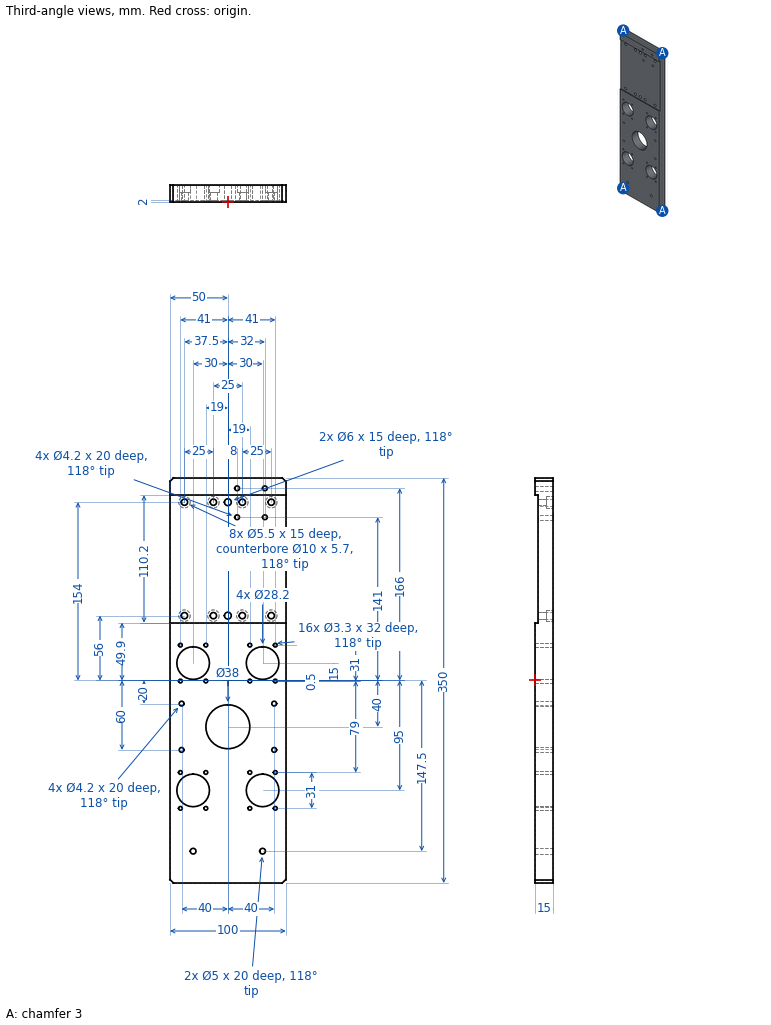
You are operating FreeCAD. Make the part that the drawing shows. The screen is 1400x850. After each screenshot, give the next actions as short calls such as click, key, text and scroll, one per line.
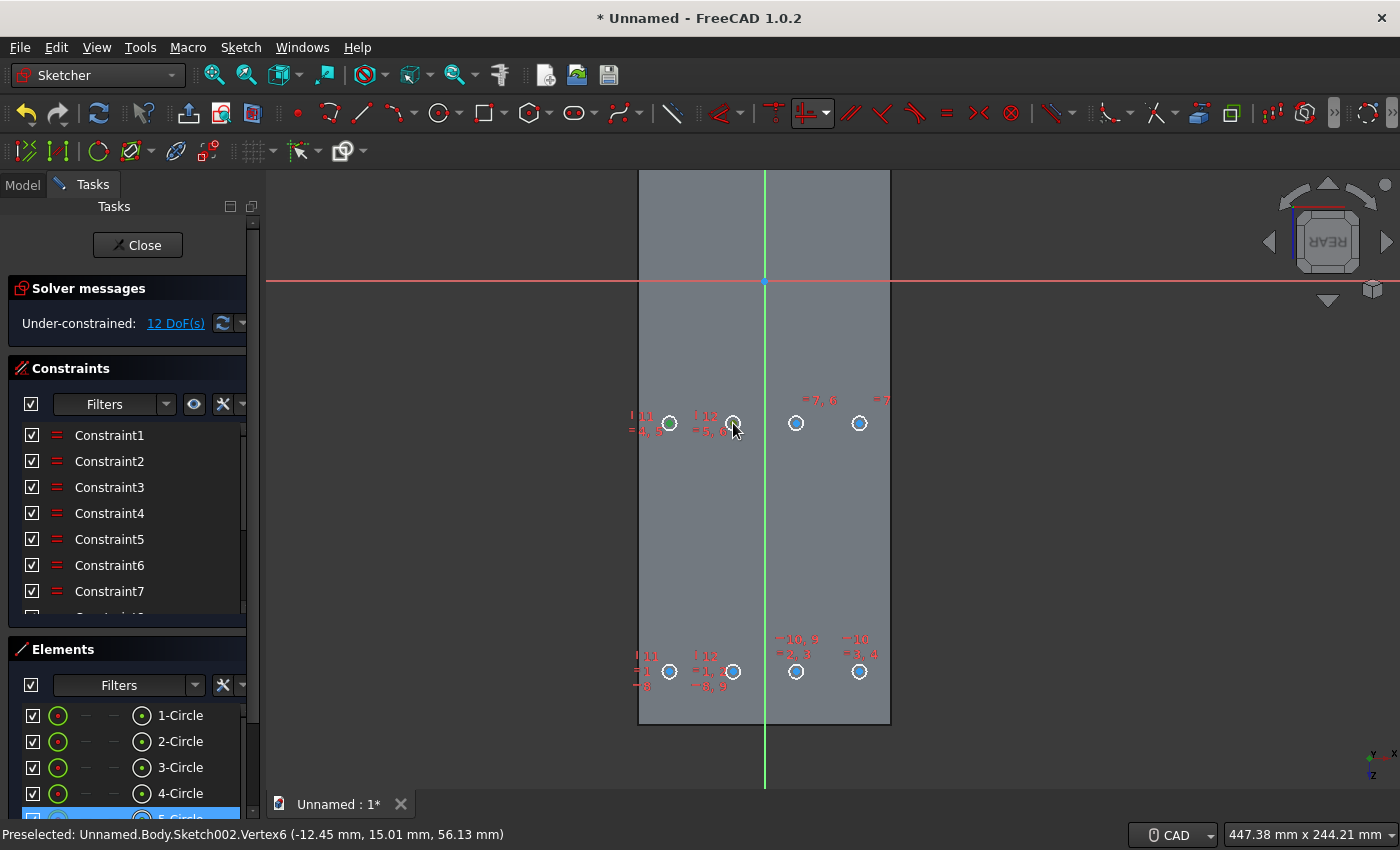
click(828, 114)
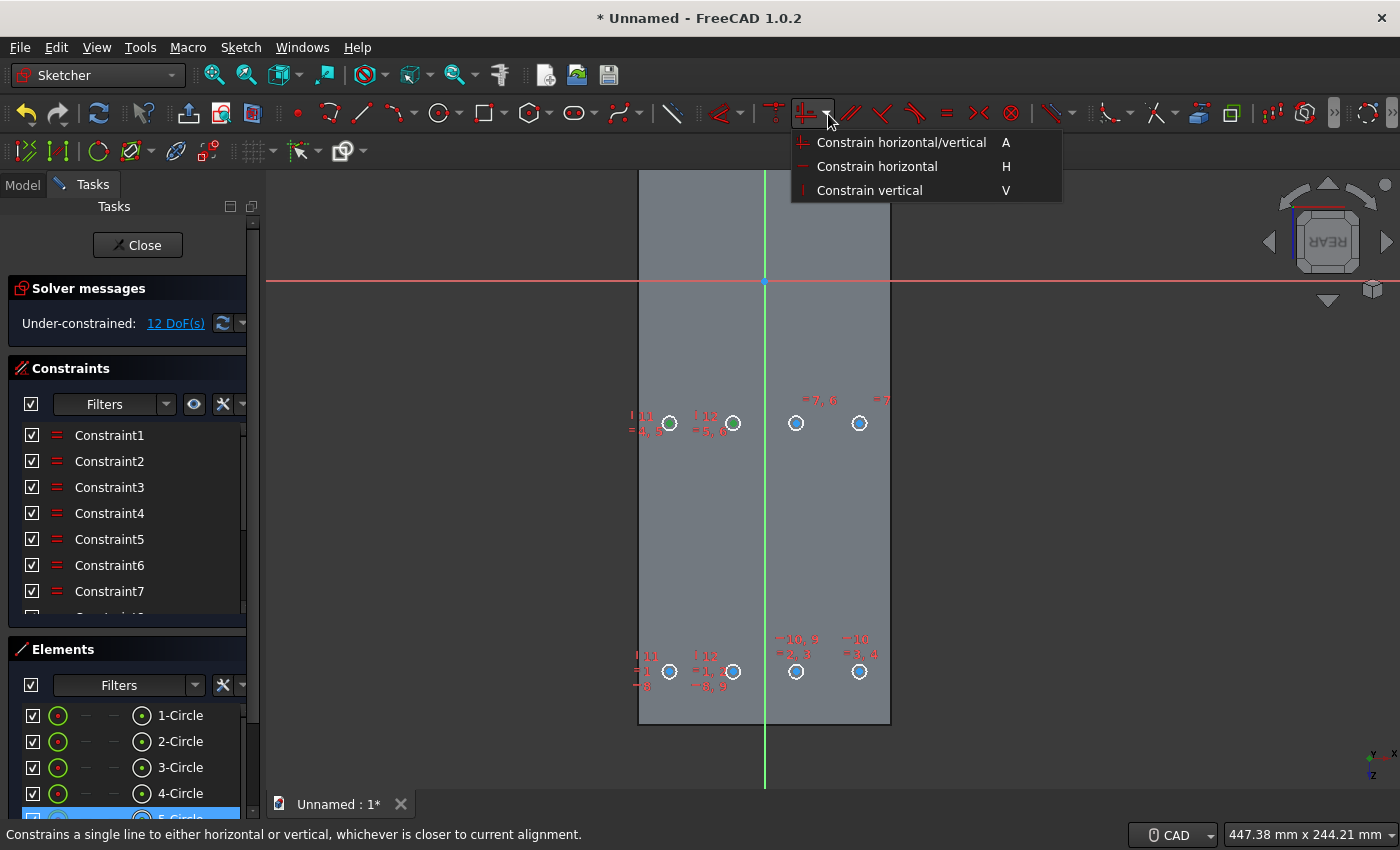
click(927, 166)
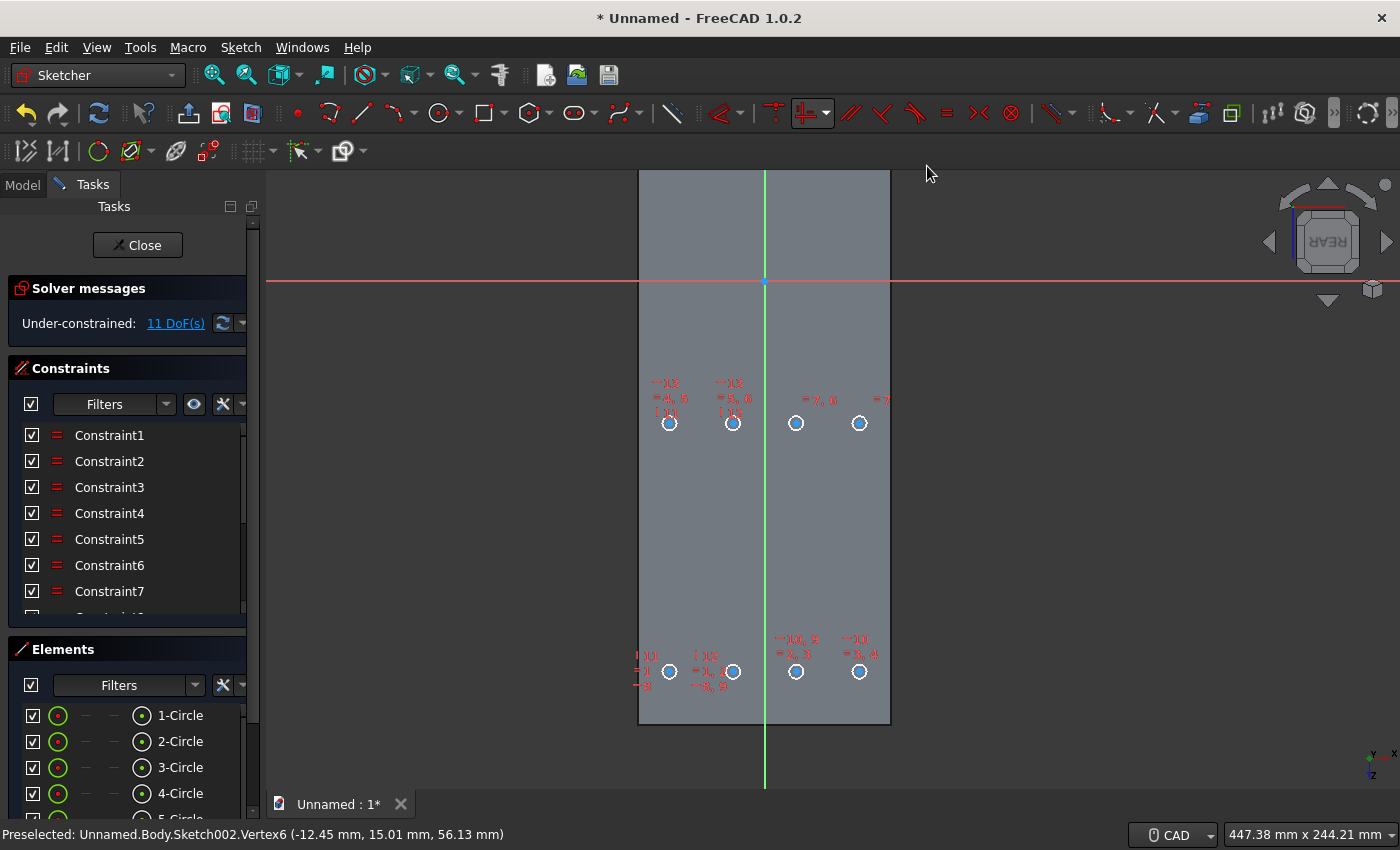
click(796, 672)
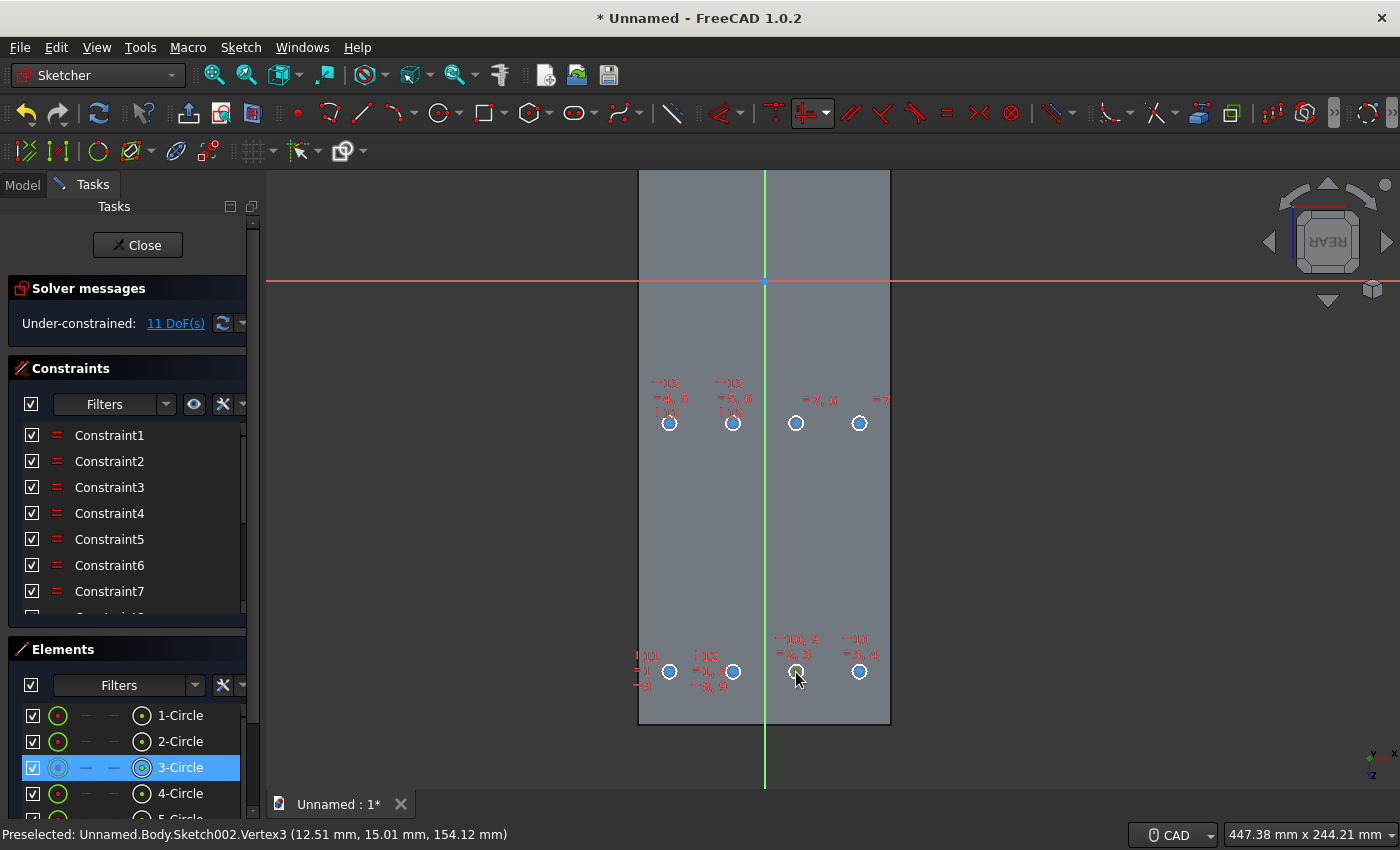
click(796, 423)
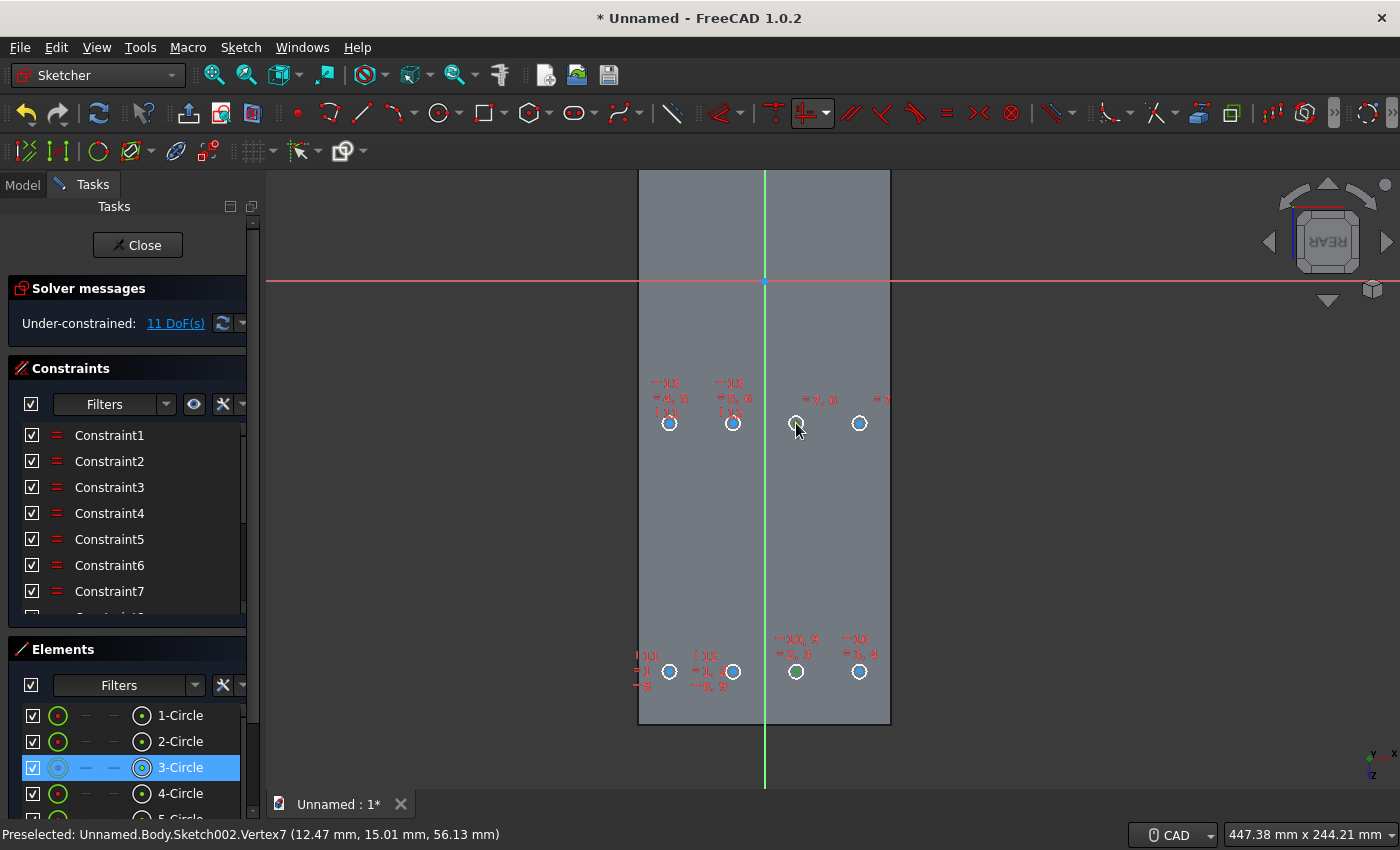
key(v)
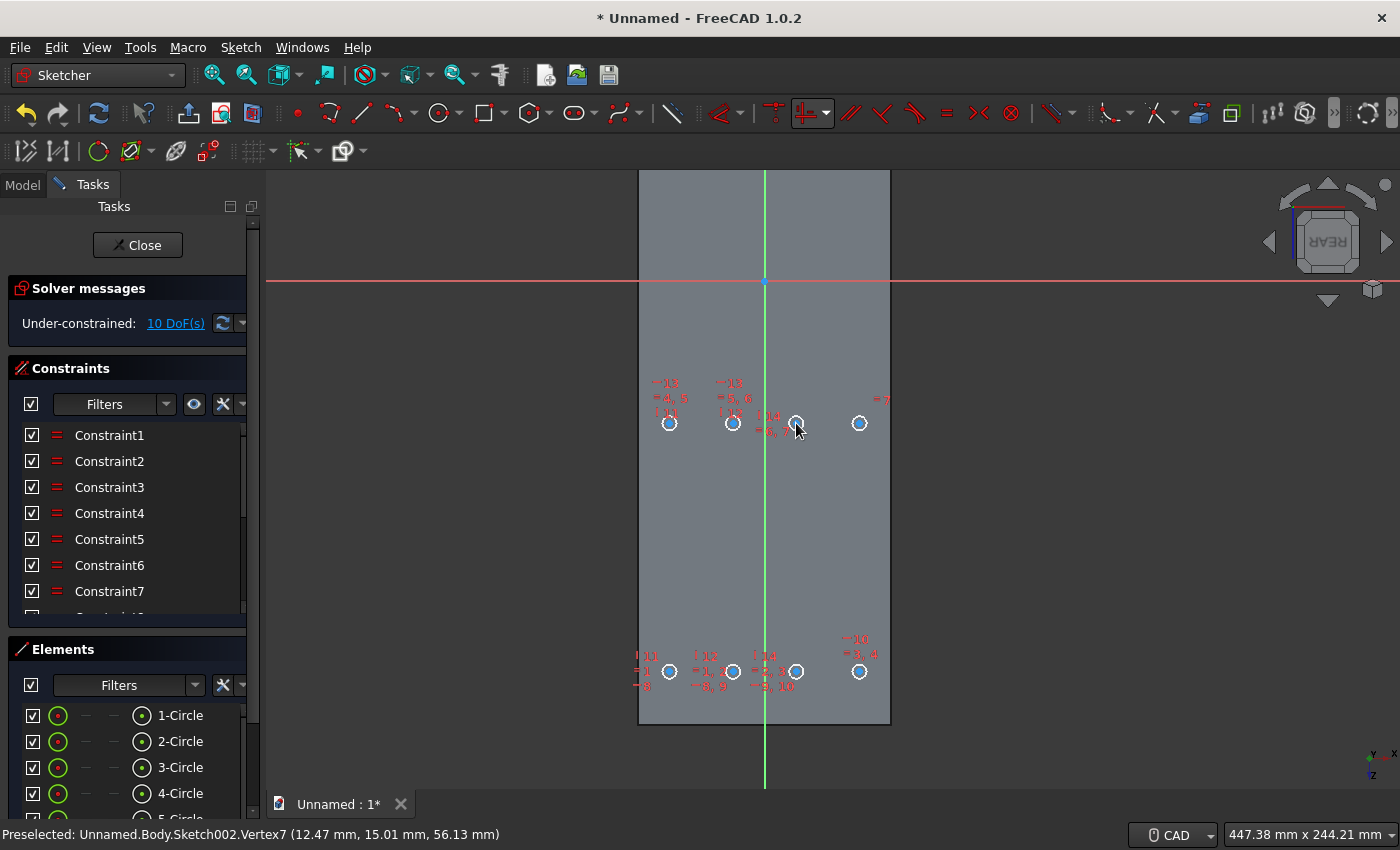
click(733, 423)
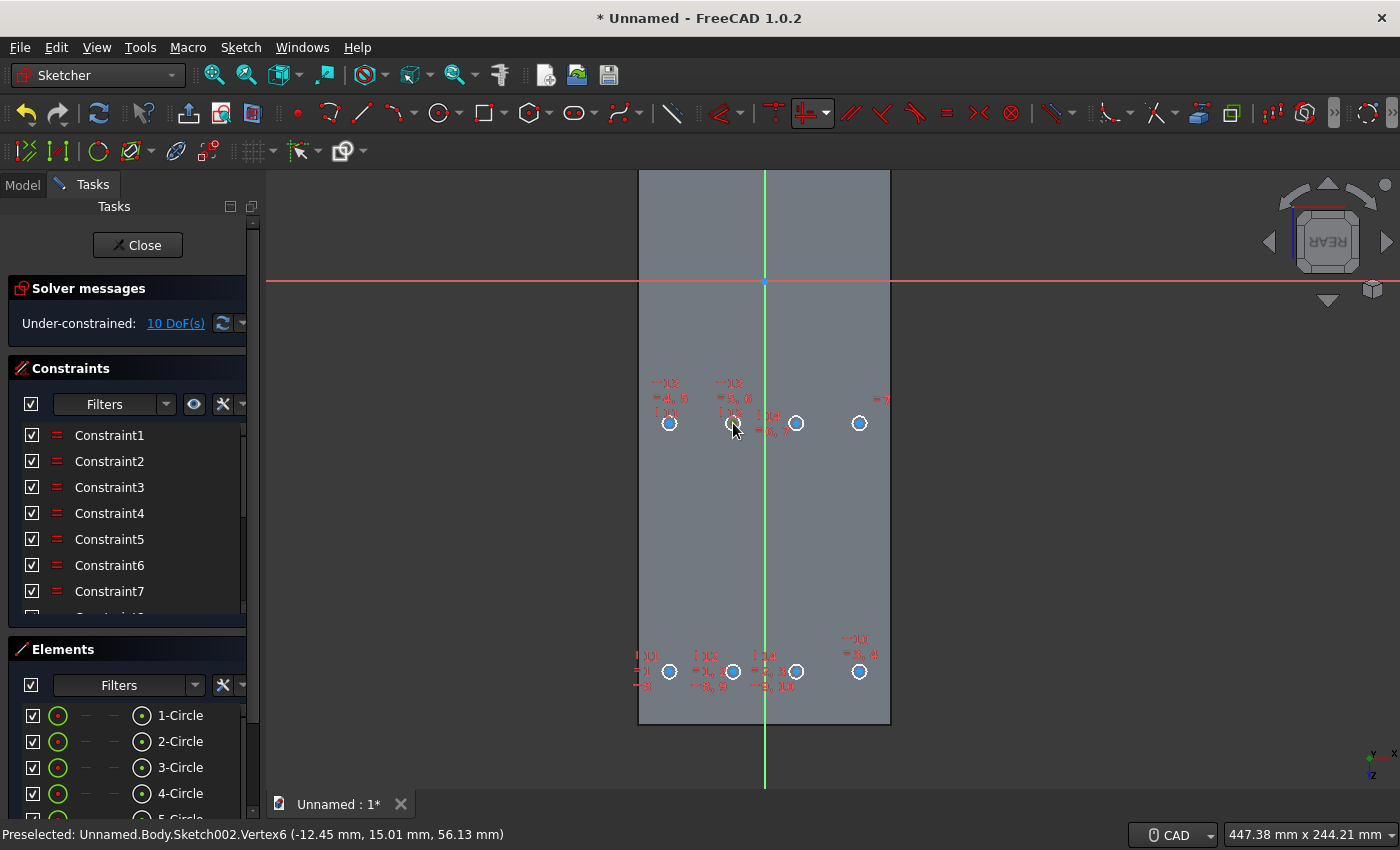
click(796, 423)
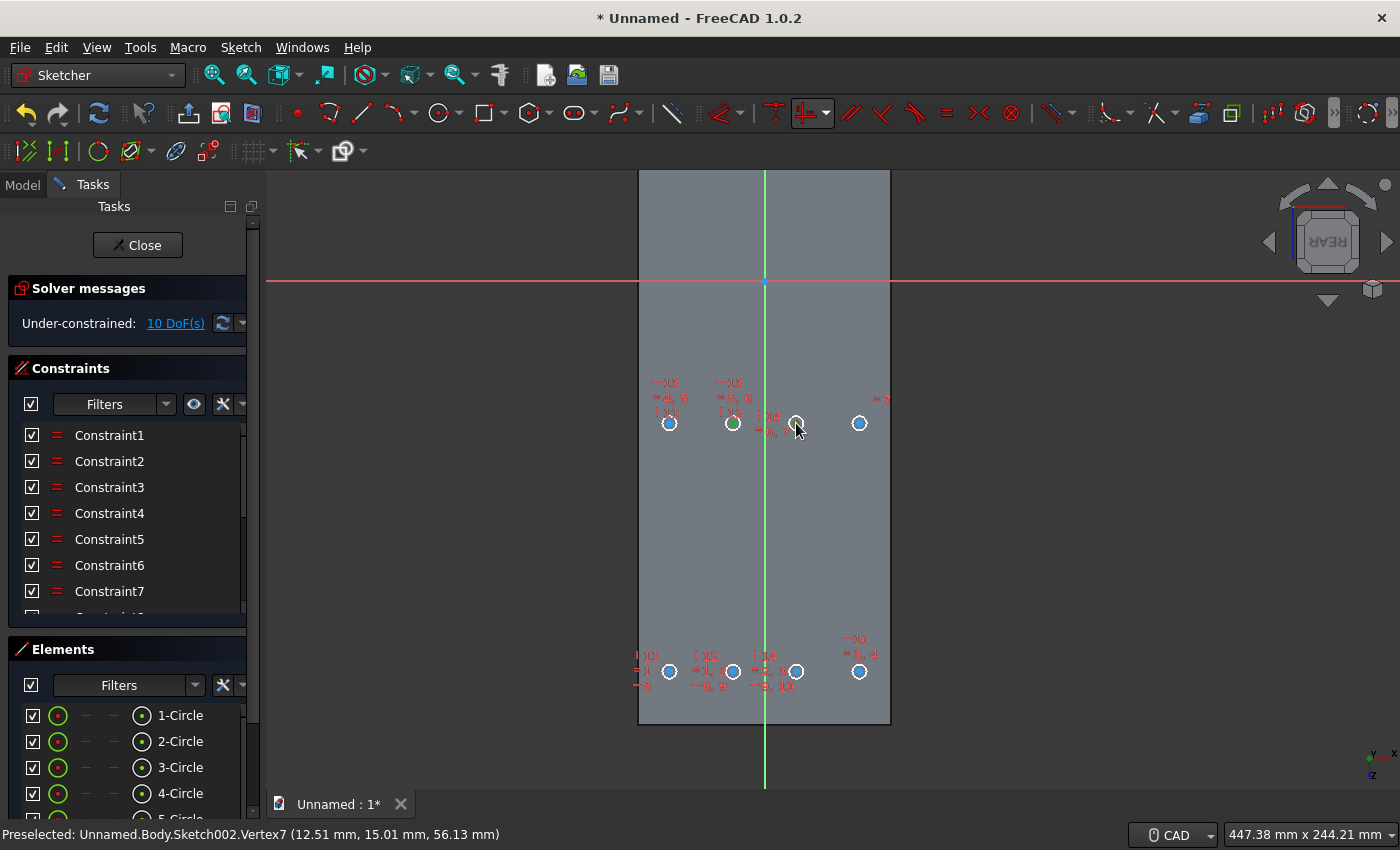
click(828, 114)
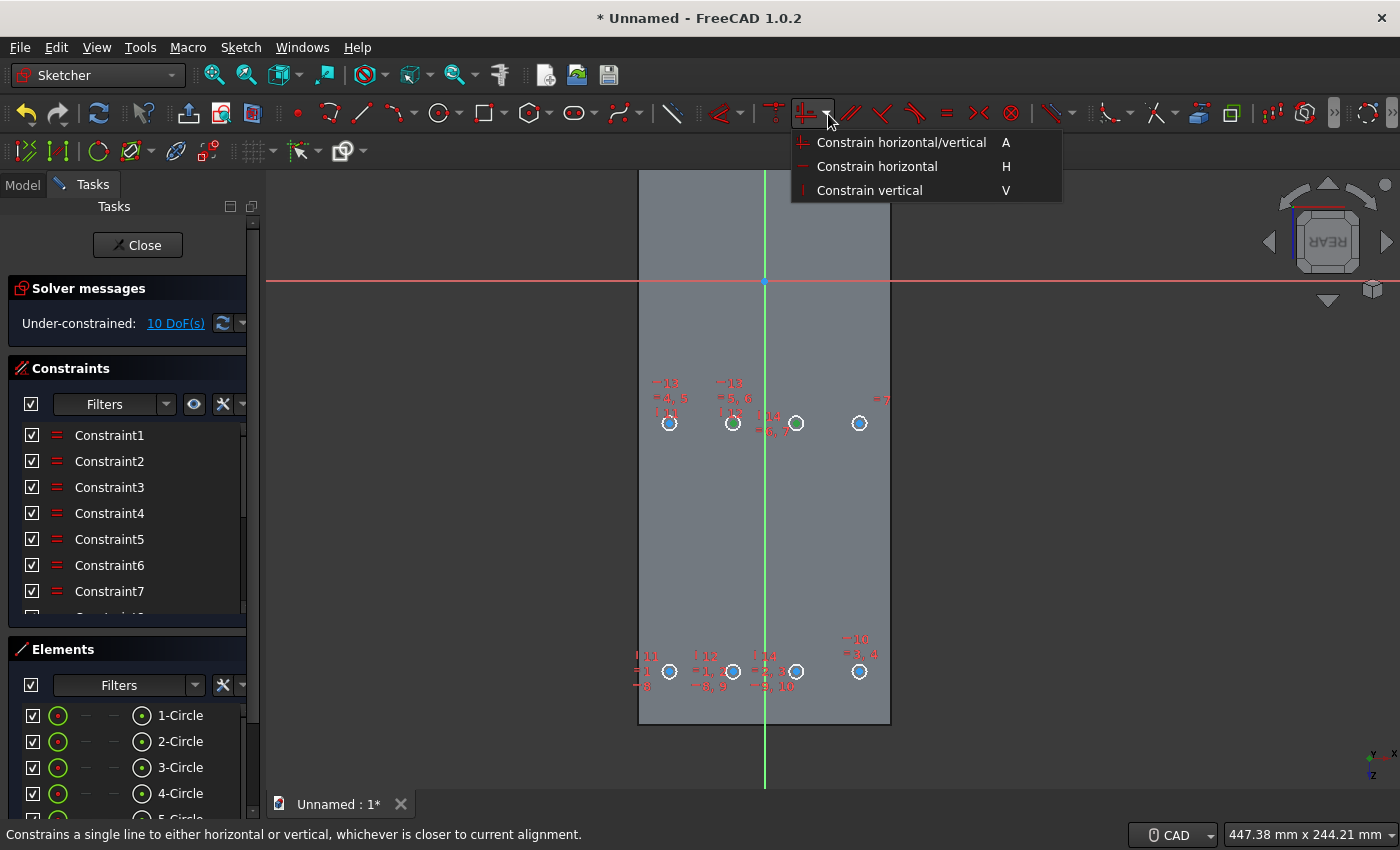
click(927, 166)